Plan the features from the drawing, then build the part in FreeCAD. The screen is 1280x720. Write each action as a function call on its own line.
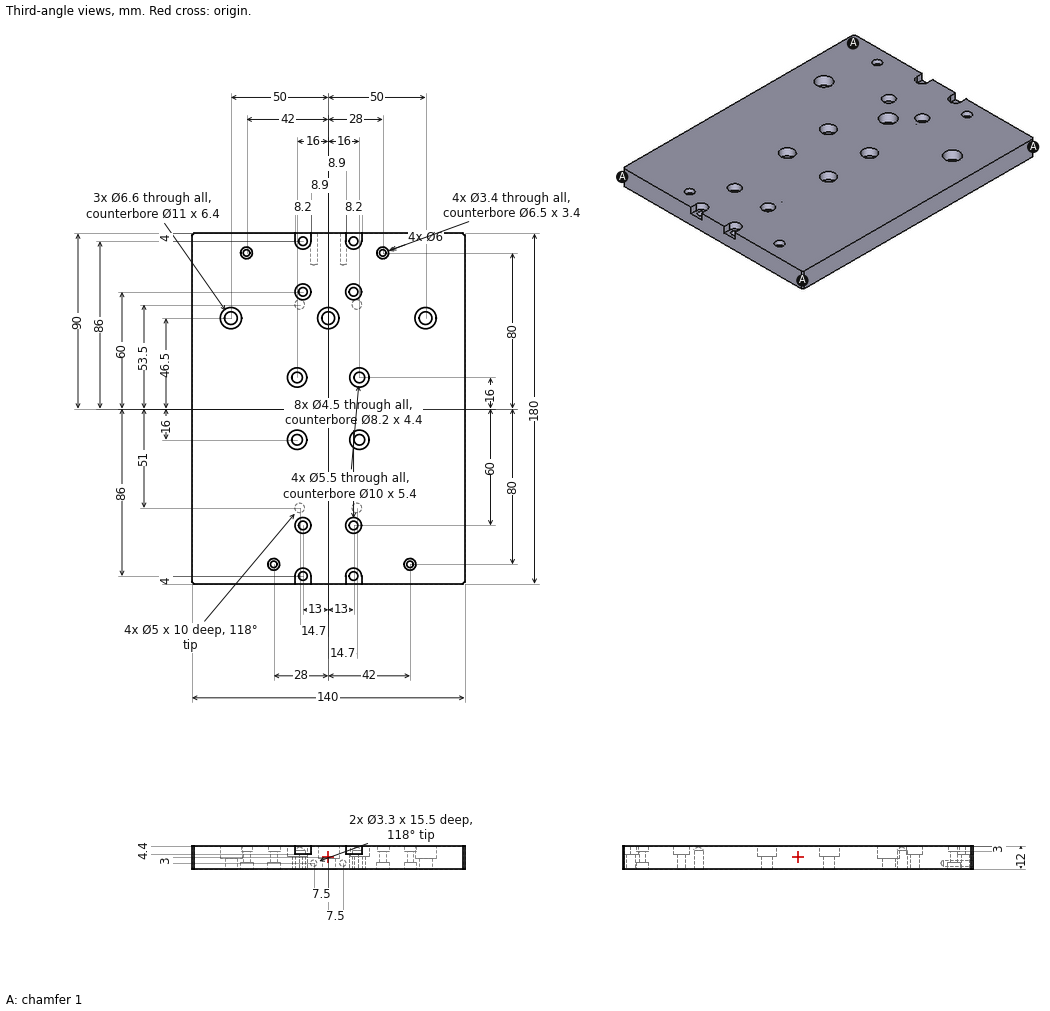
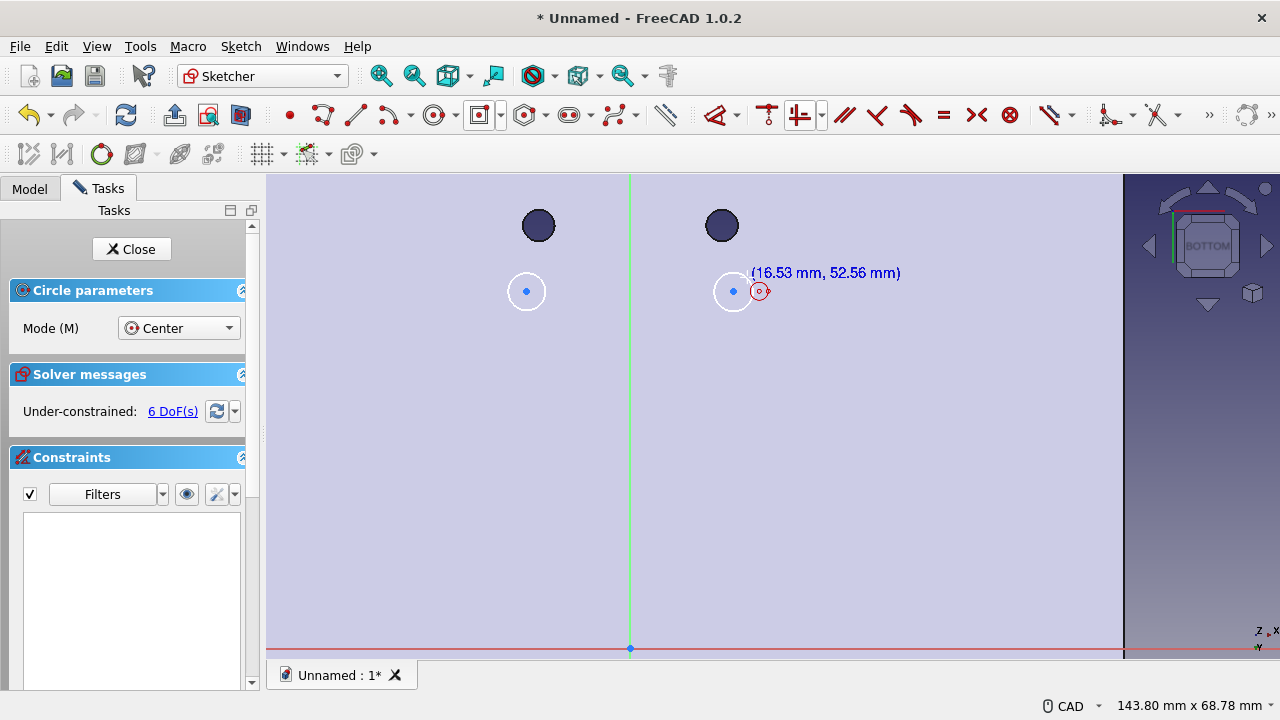
scroll(748, 276, down, 5)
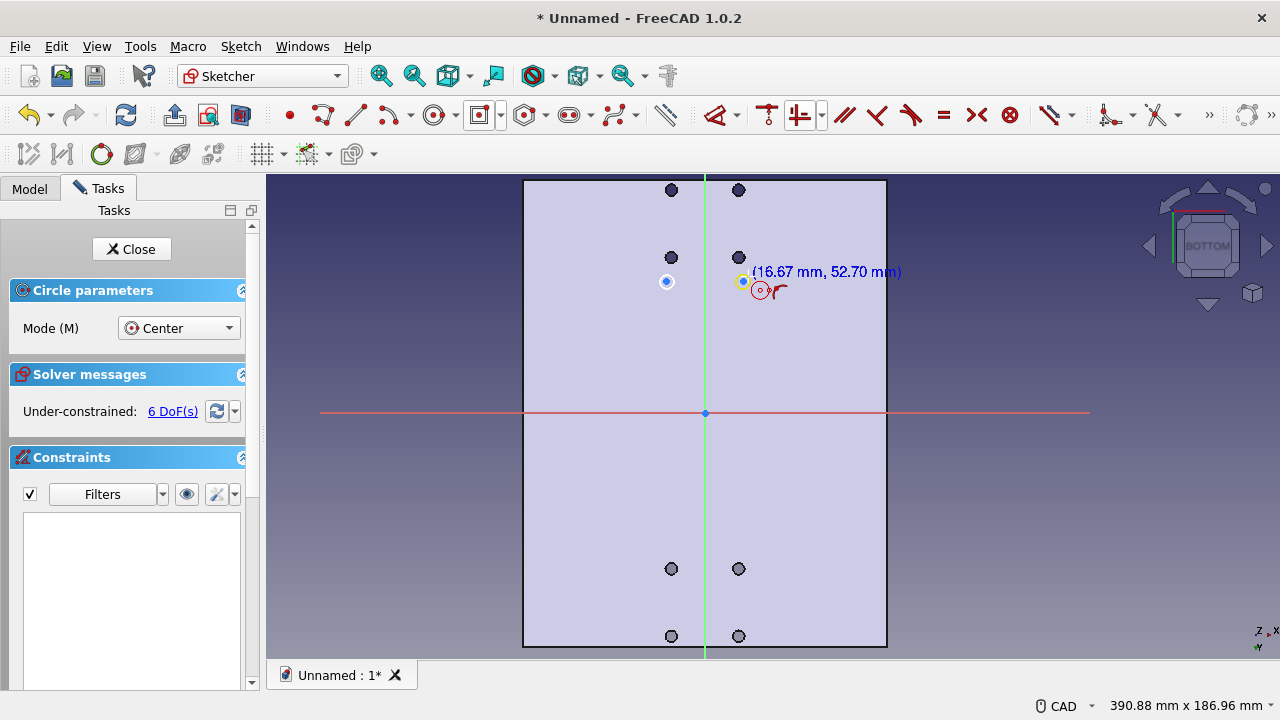
scroll(667, 552, up, 7)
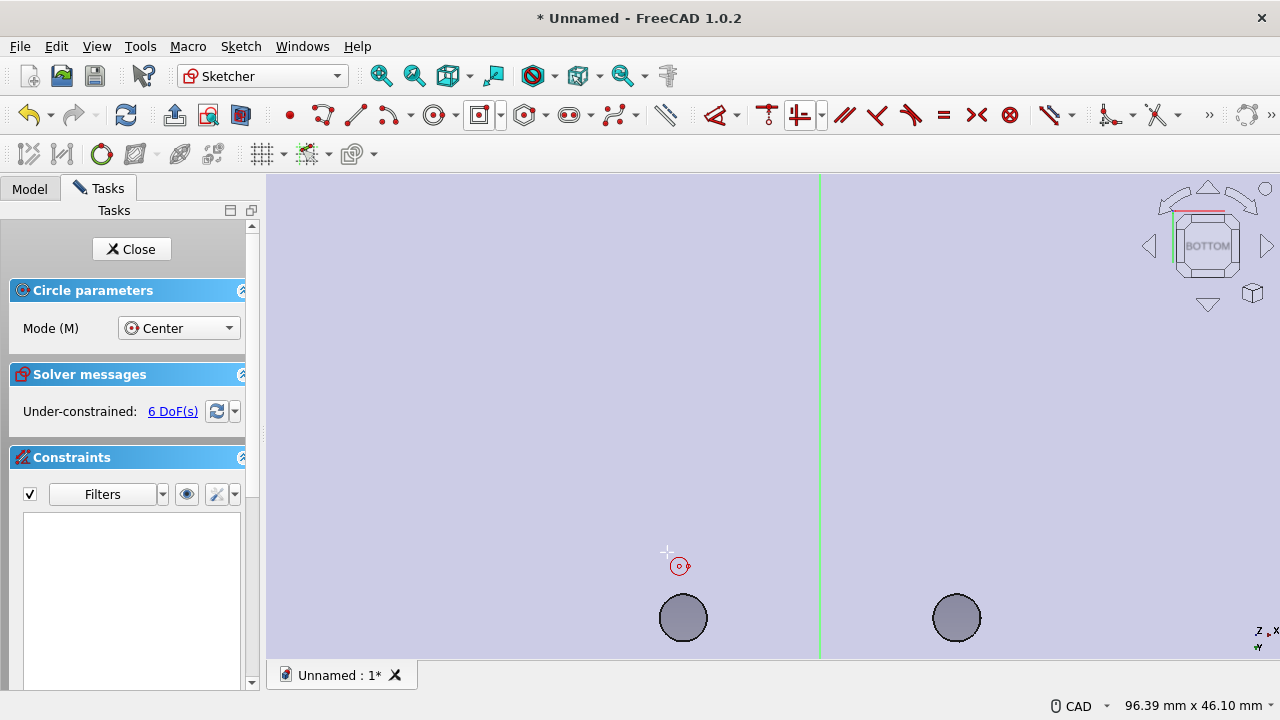
scroll(667, 553, down, 7)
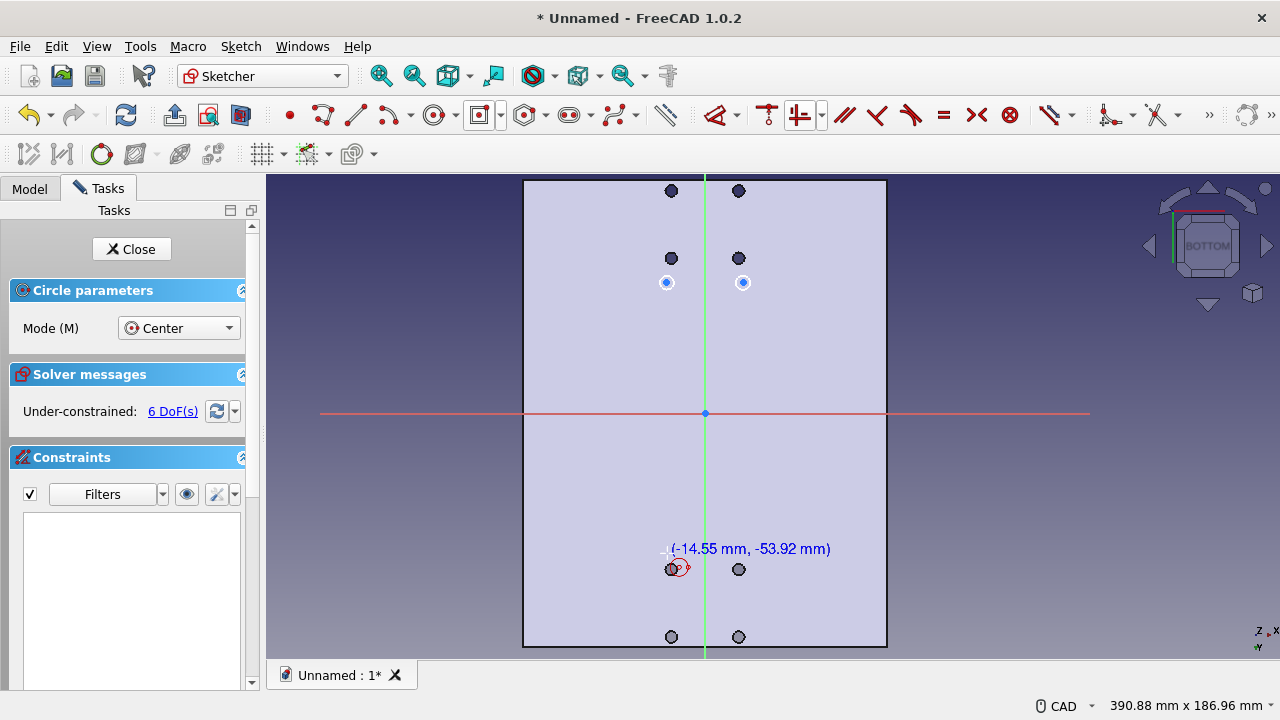
click(667, 553)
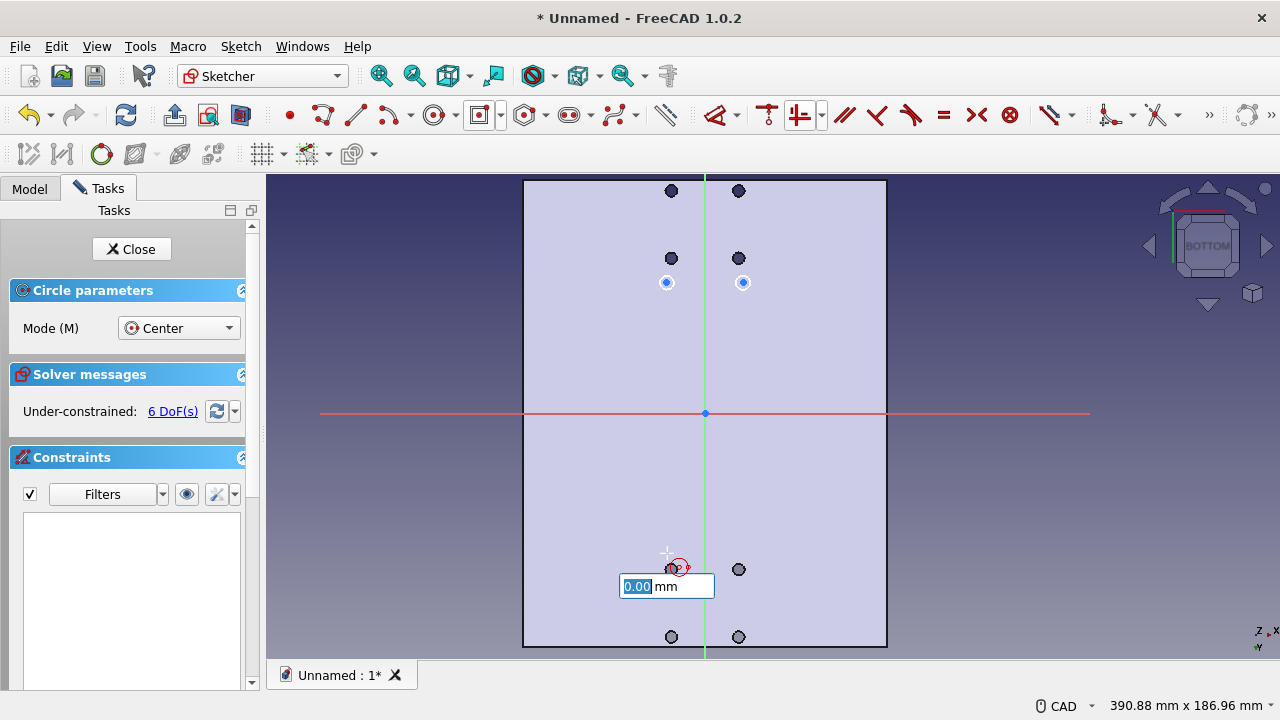
scroll(671, 548, up, 5)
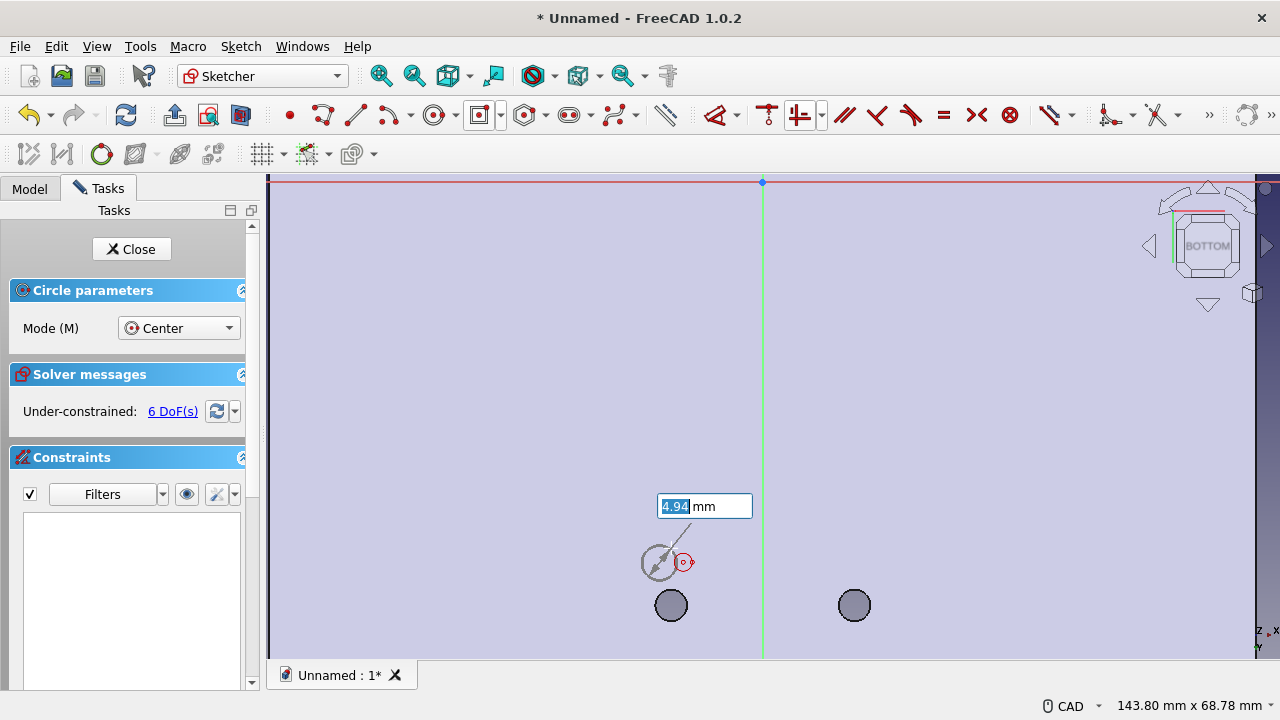
click(672, 547)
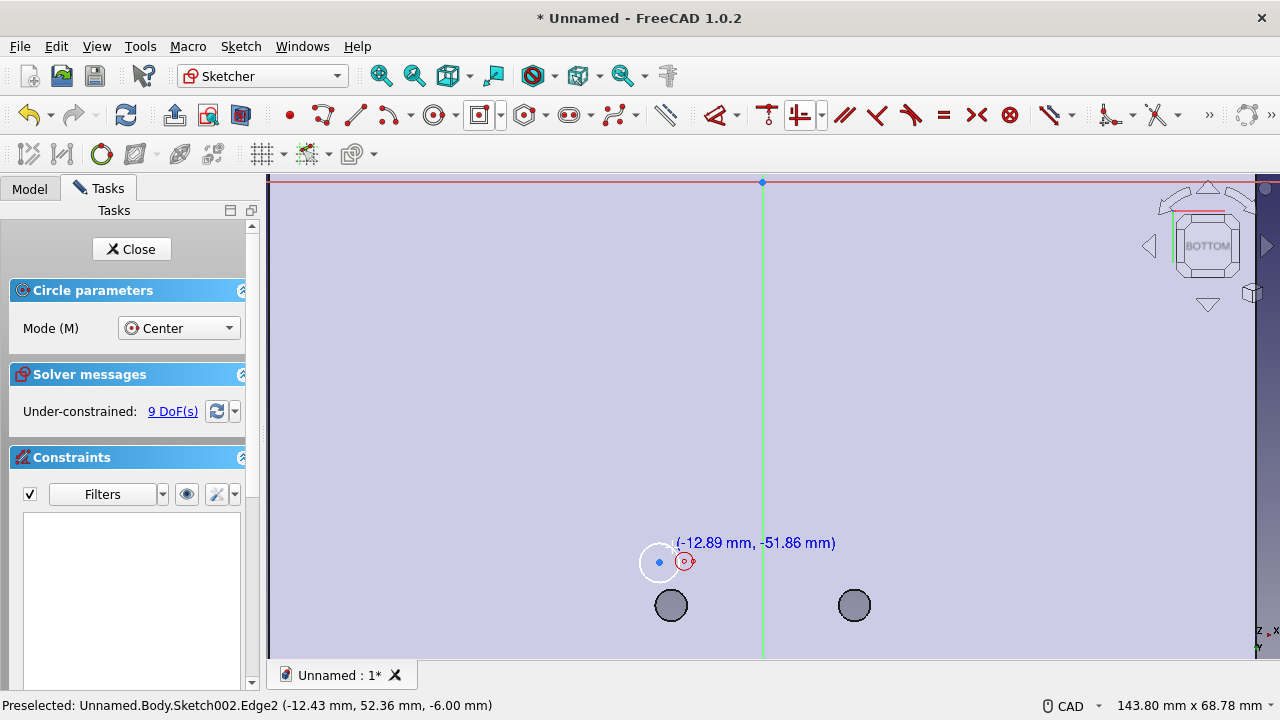
scroll(867, 560, up, 2)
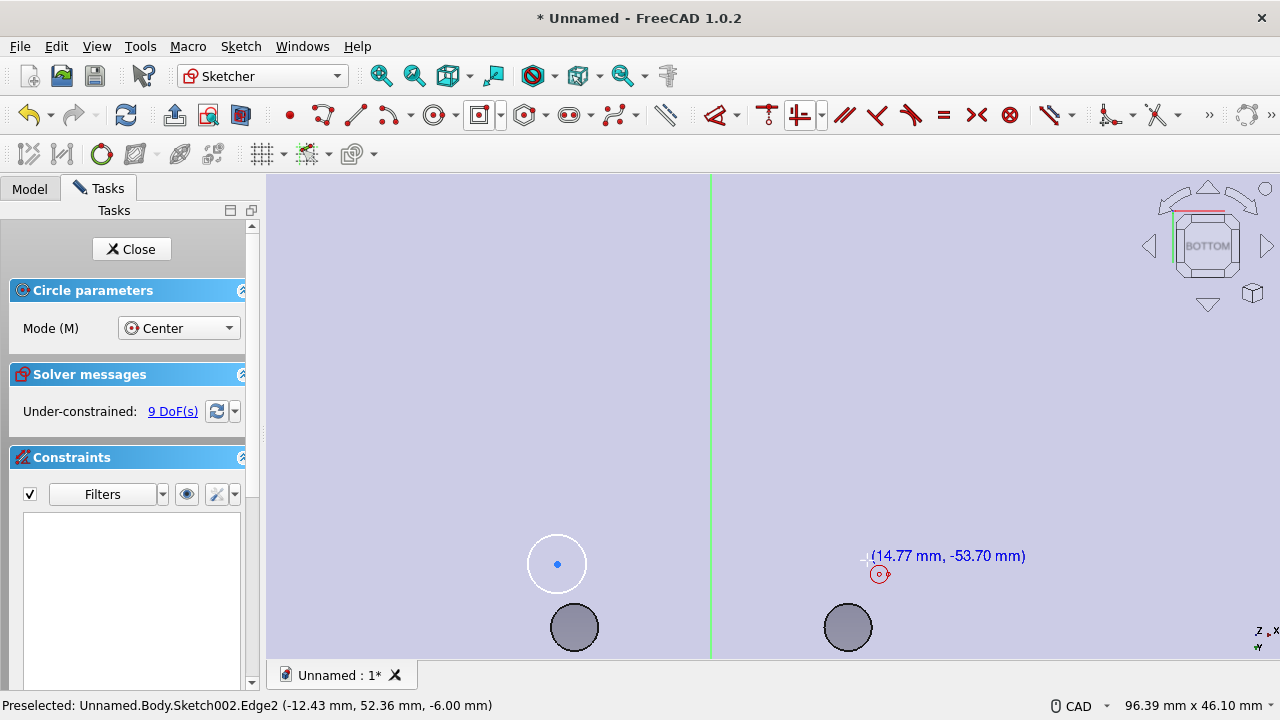
scroll(702, 550, down, 7)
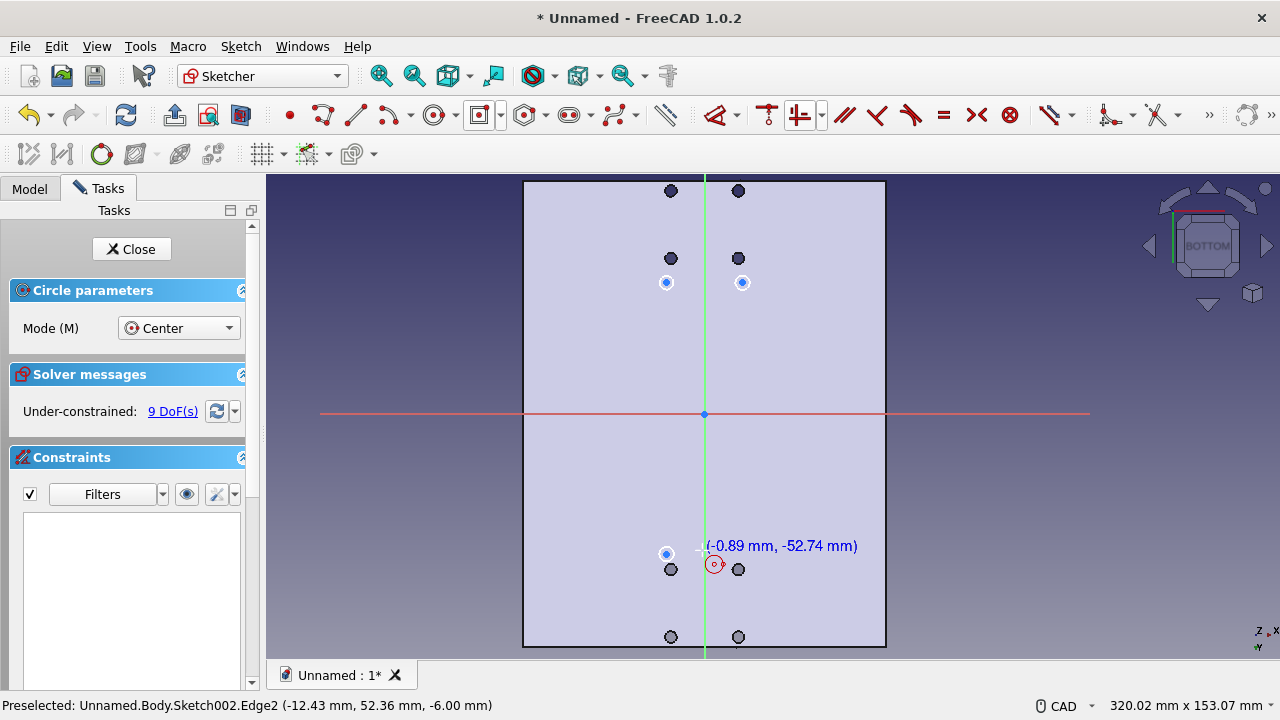
click(743, 553)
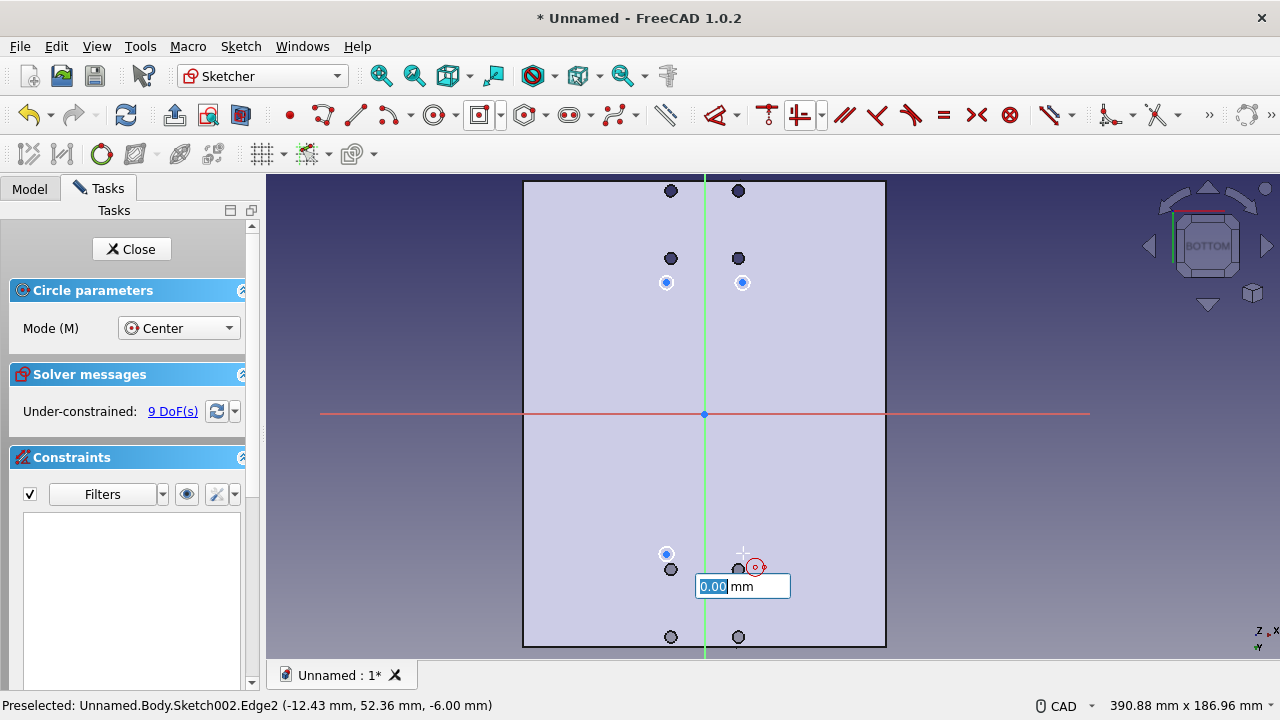
scroll(747, 548, up, 5)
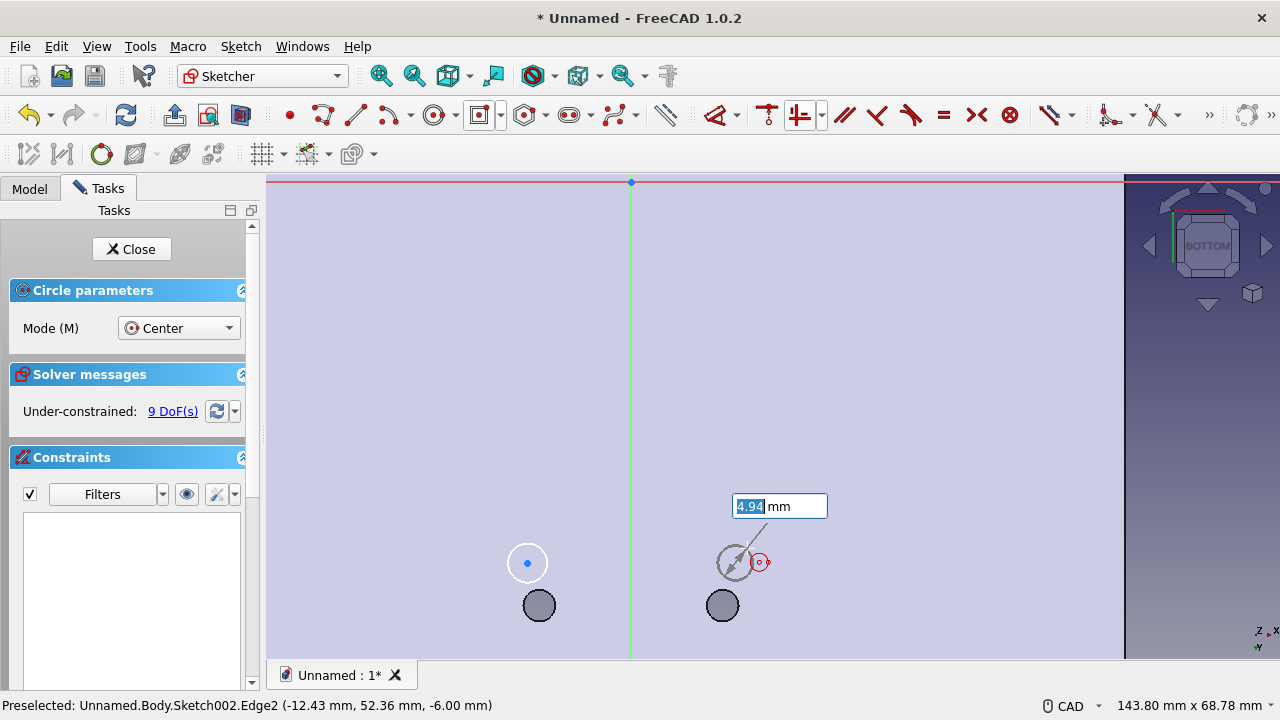
click(747, 547)
key(Escape)